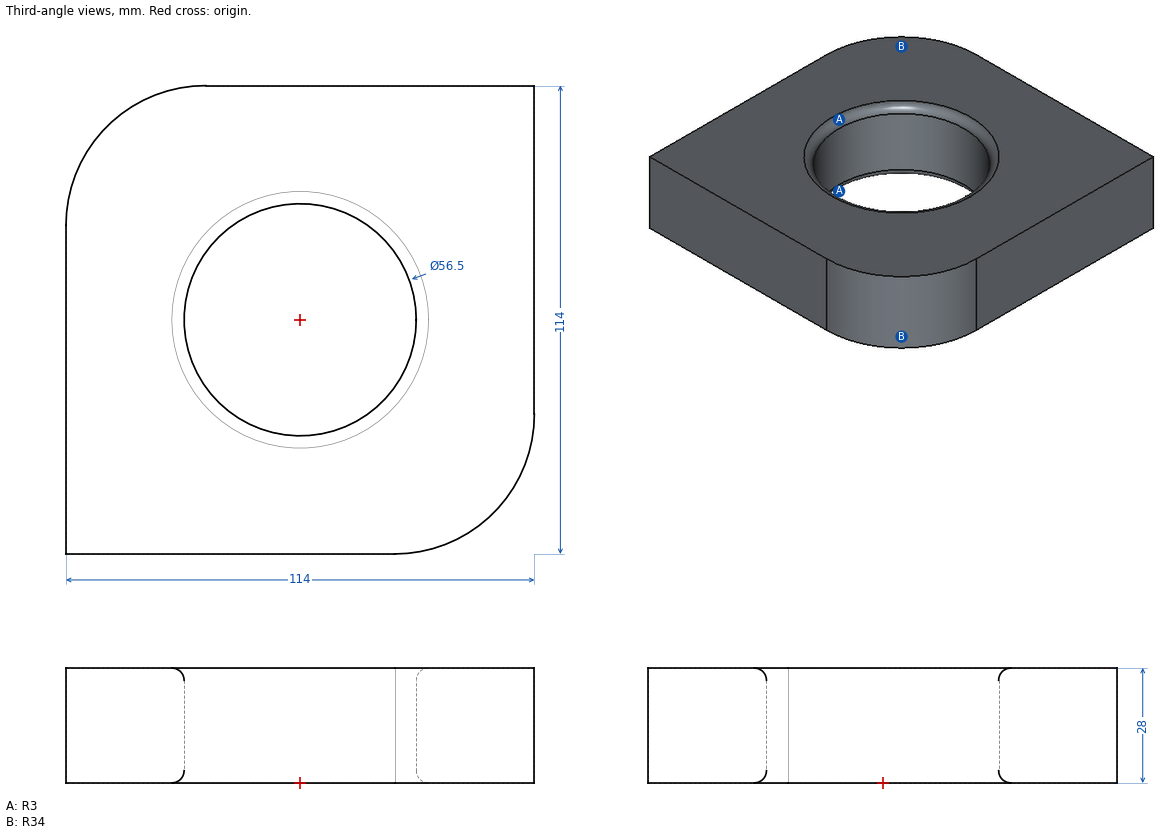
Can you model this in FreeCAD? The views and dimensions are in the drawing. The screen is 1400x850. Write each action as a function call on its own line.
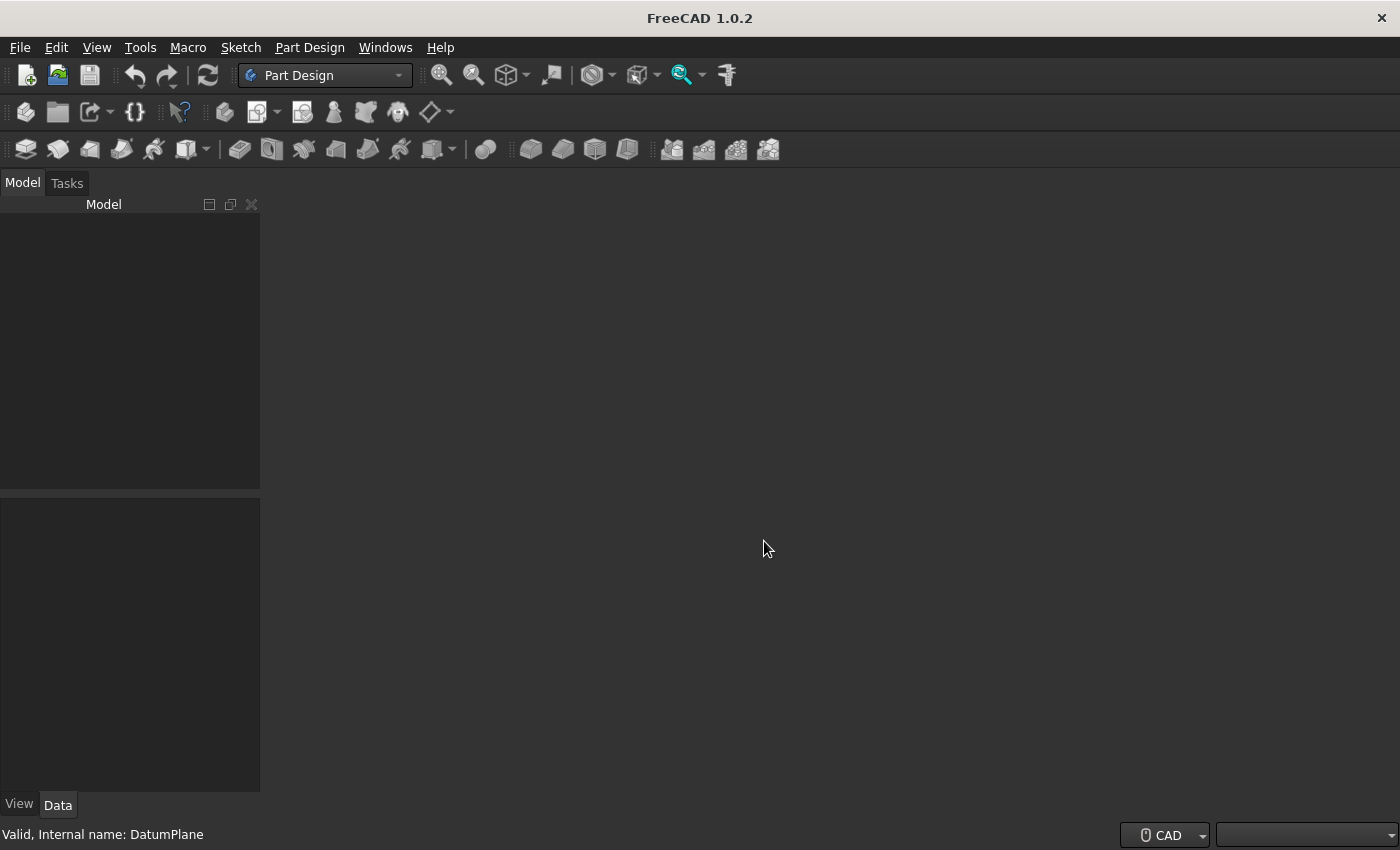
key(ctrl+n)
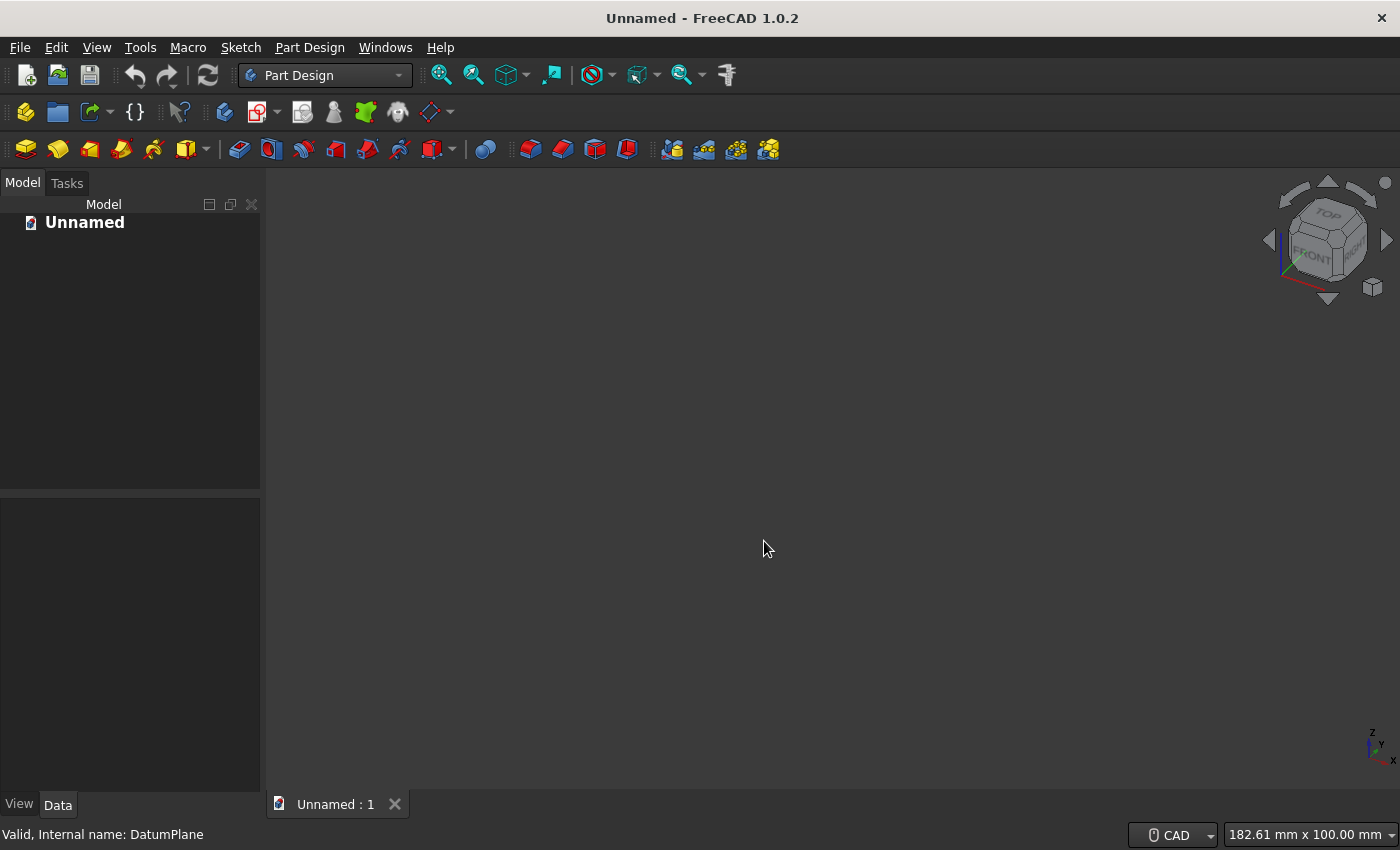
click(258, 112)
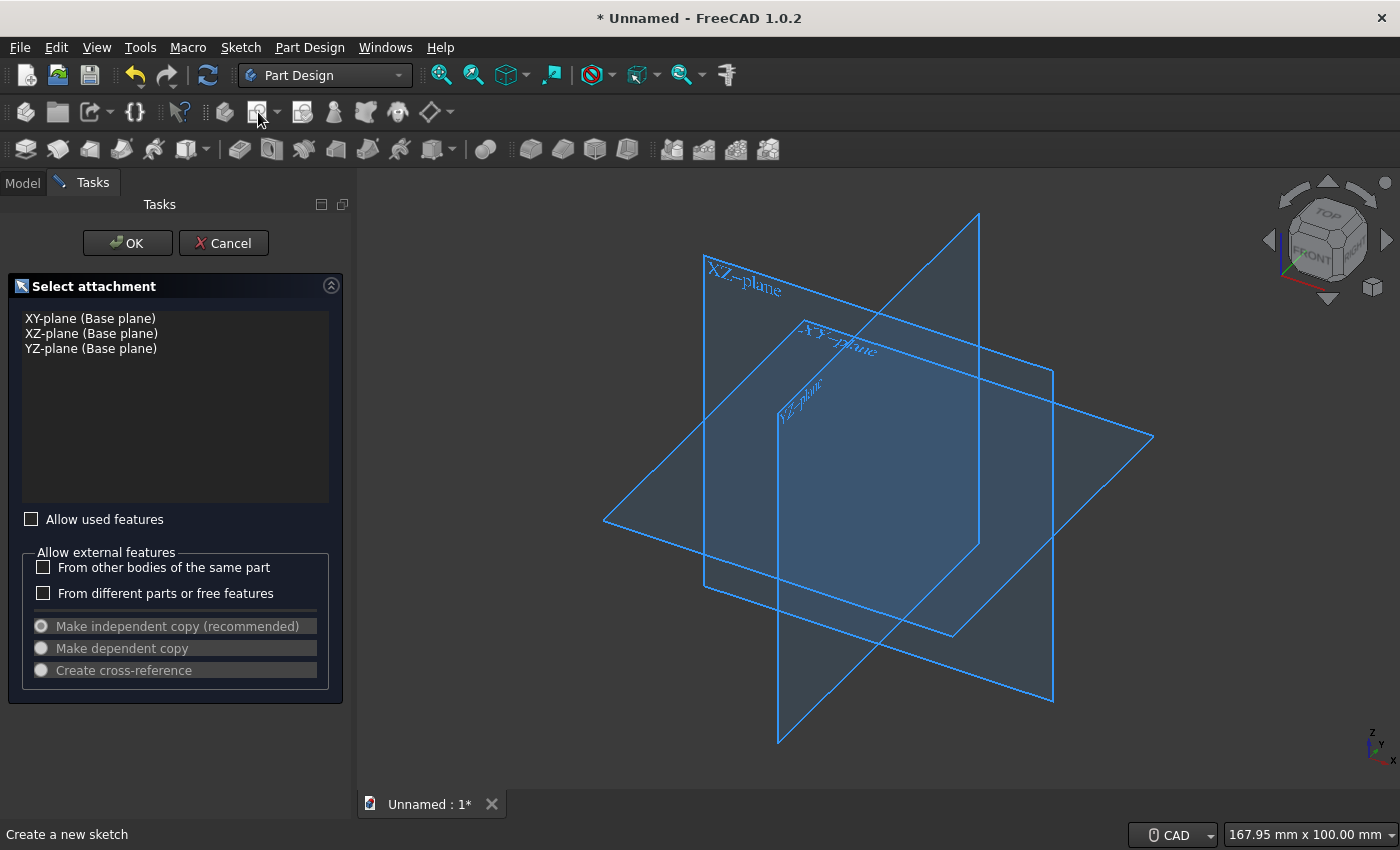
click(82, 318)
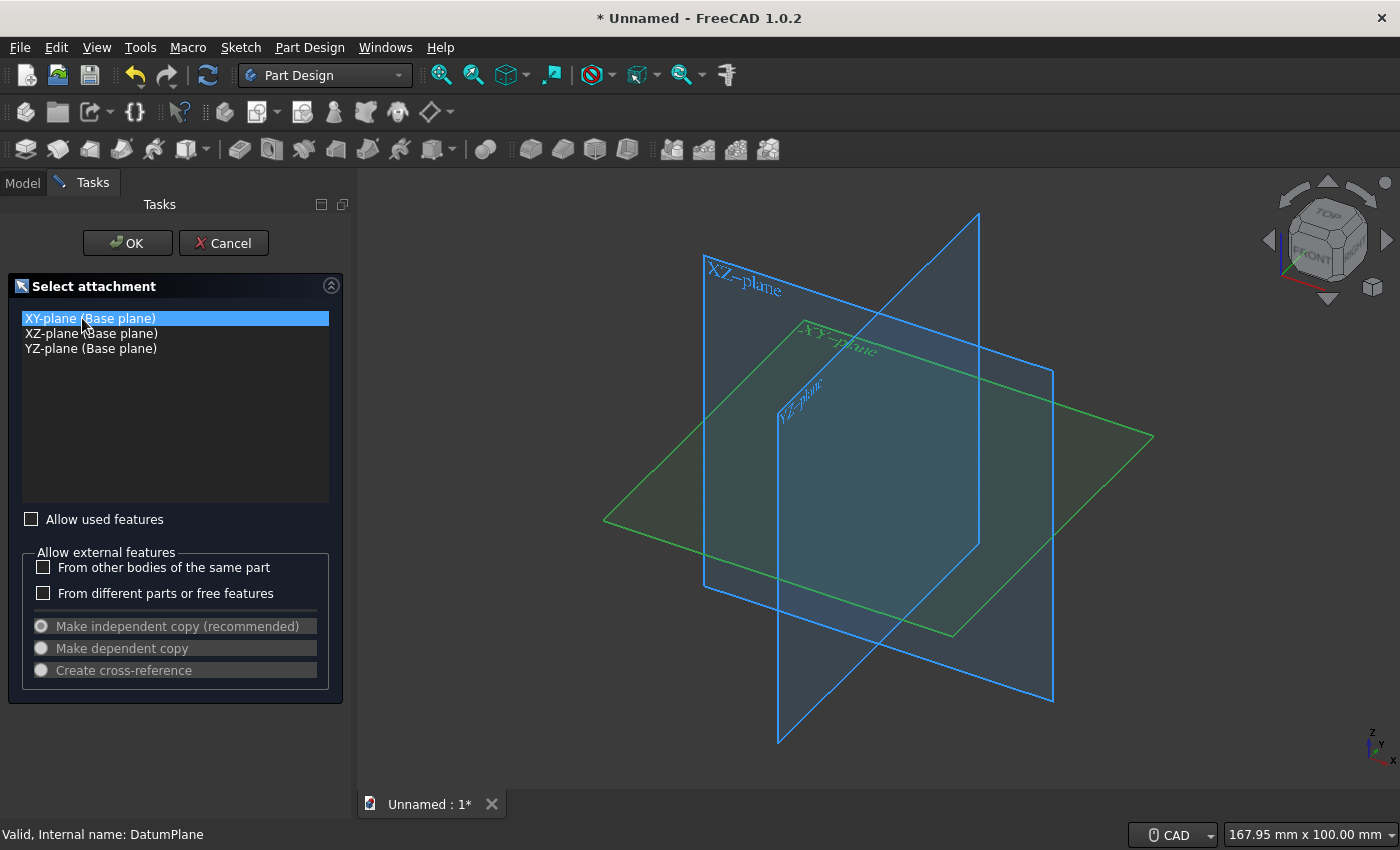
click(128, 243)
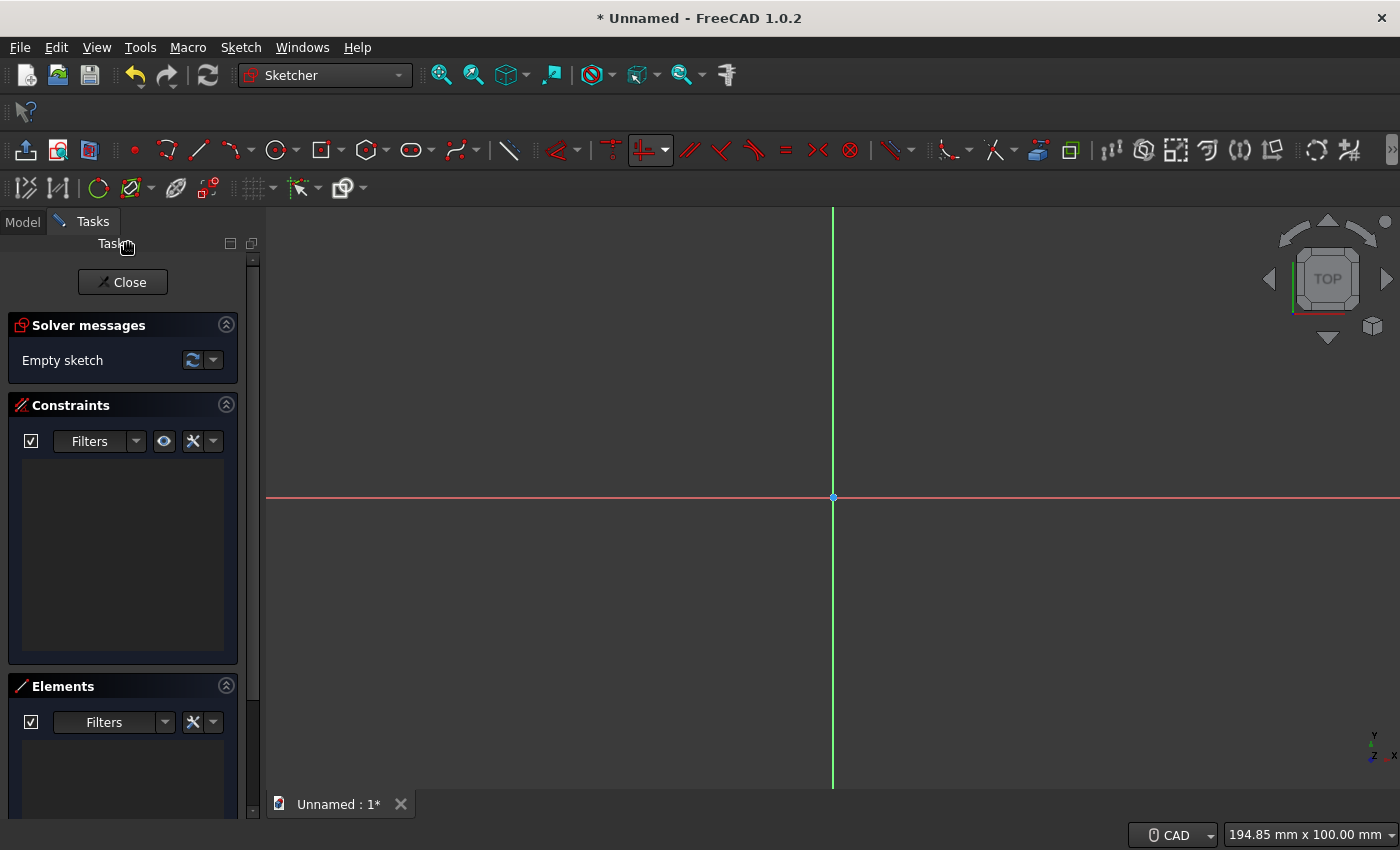
scroll(681, 498, down, 3)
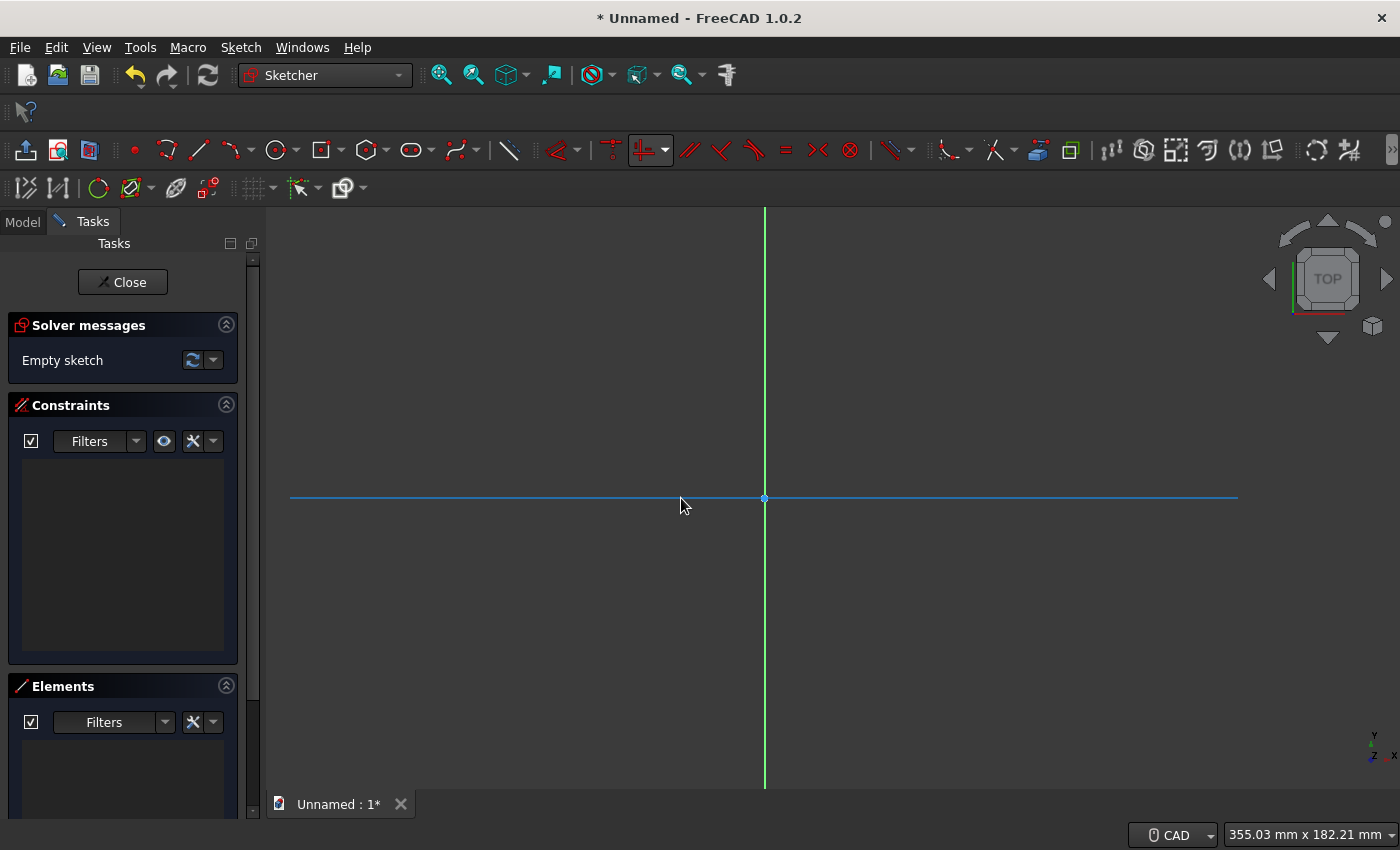
click(322, 150)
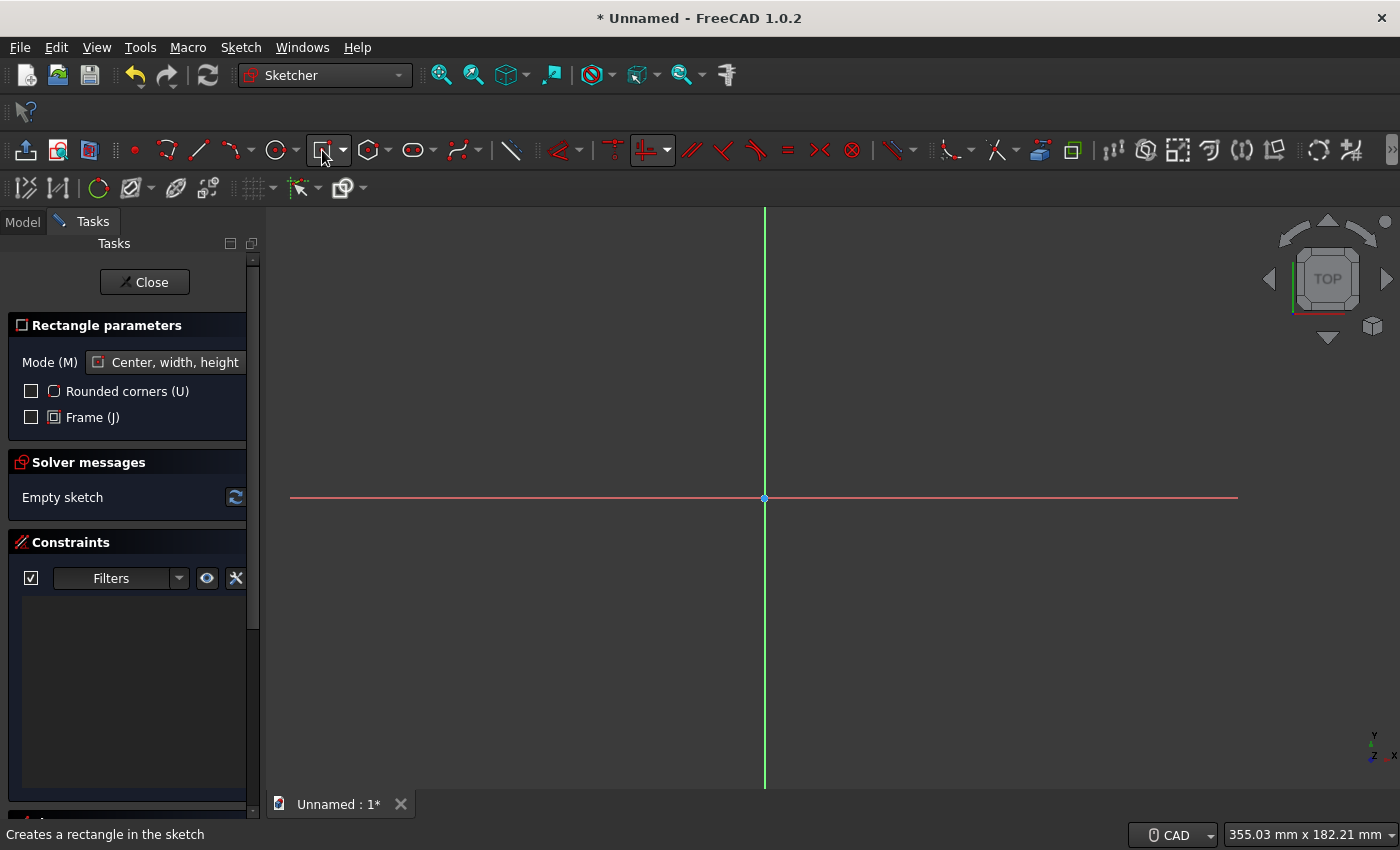
click(765, 498)
click(947, 316)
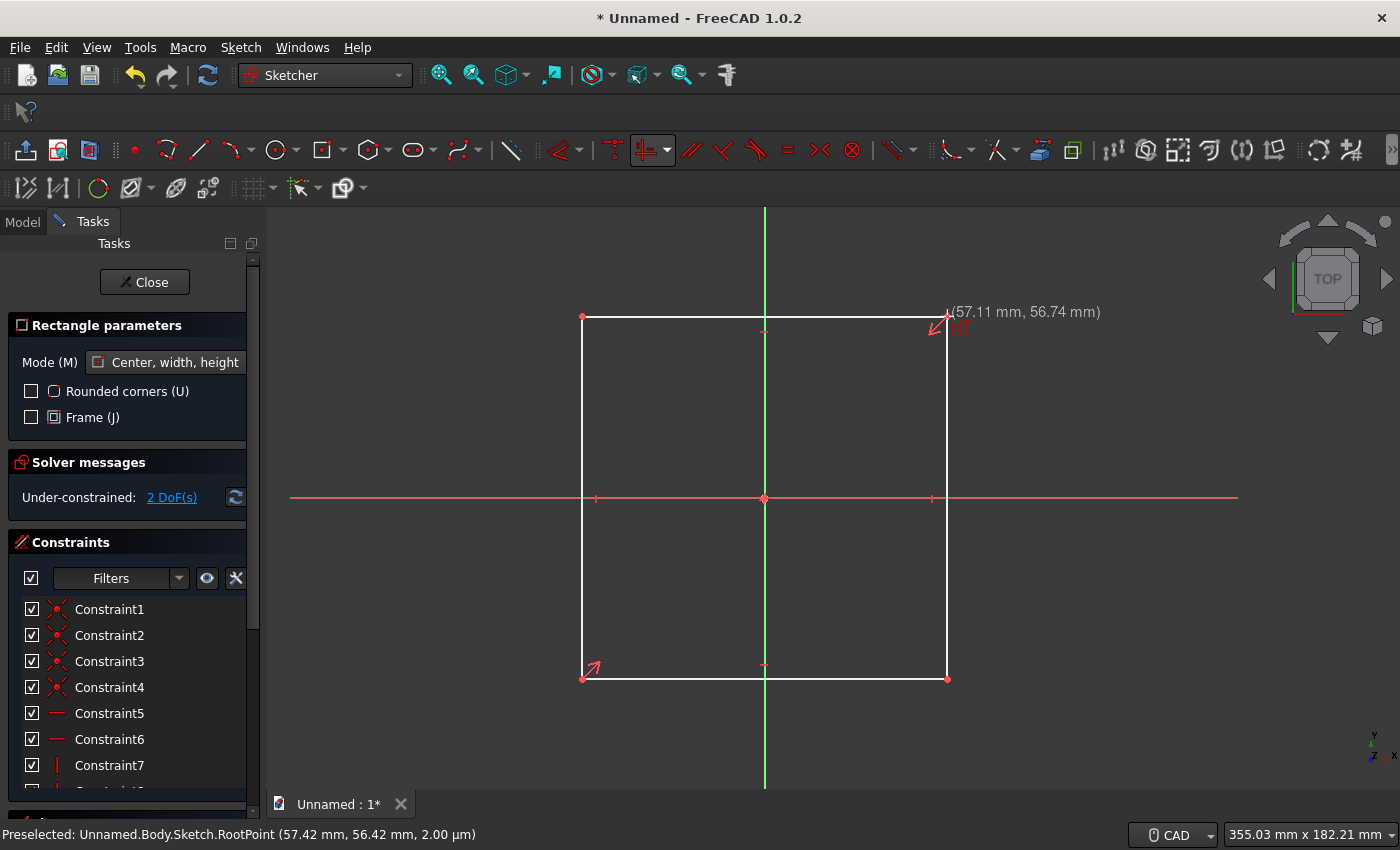
key(g)
key(c)